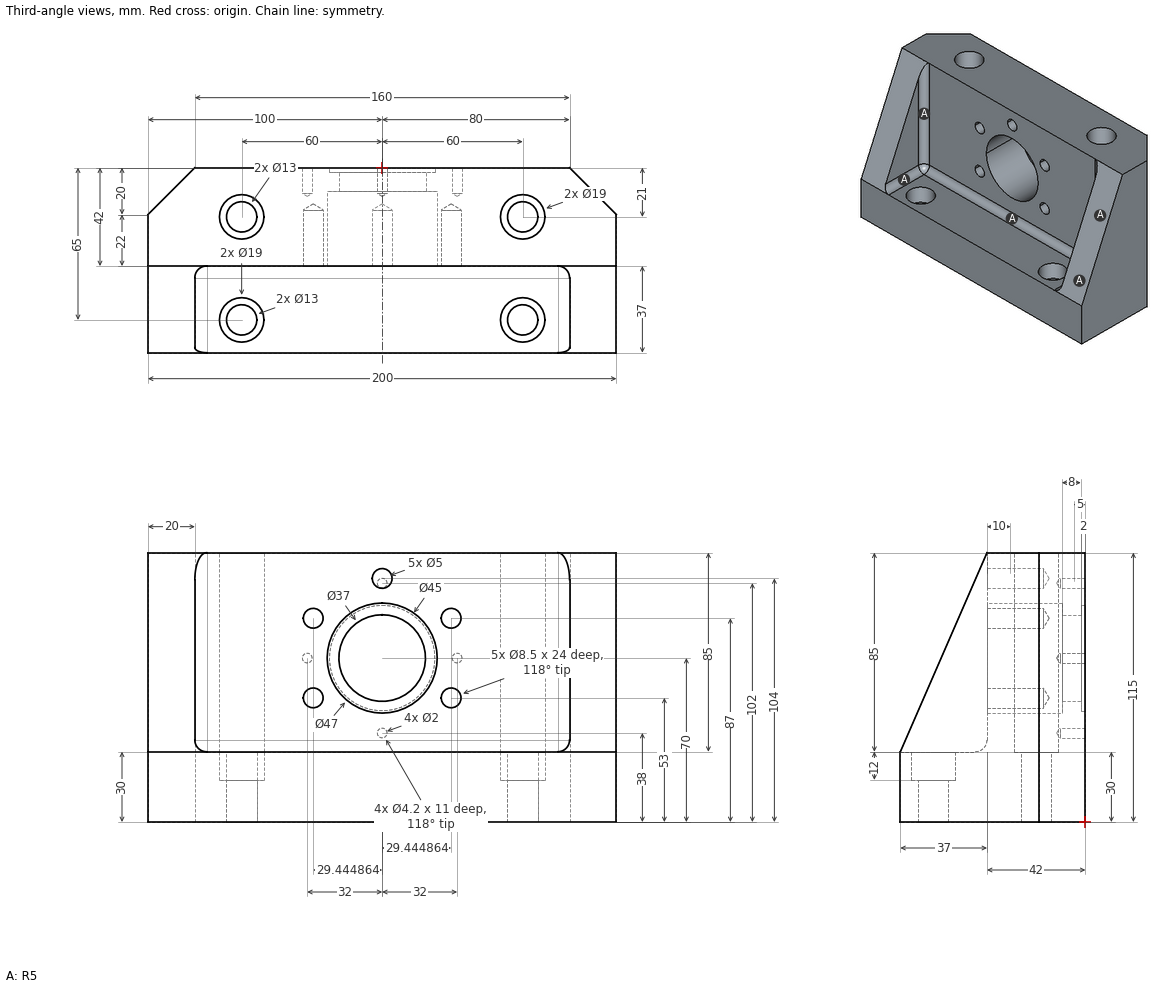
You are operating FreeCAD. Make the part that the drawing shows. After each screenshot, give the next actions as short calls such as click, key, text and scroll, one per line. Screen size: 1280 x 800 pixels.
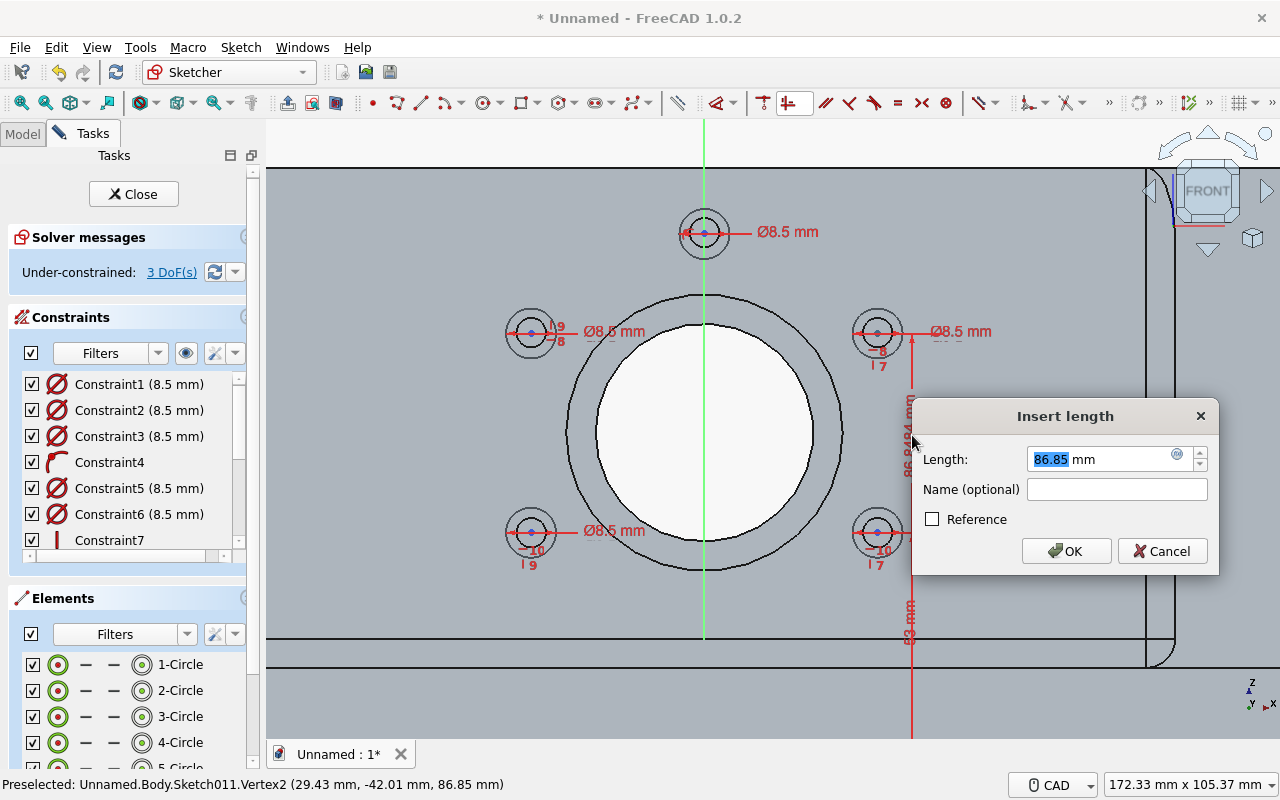
text(87)
key(Return)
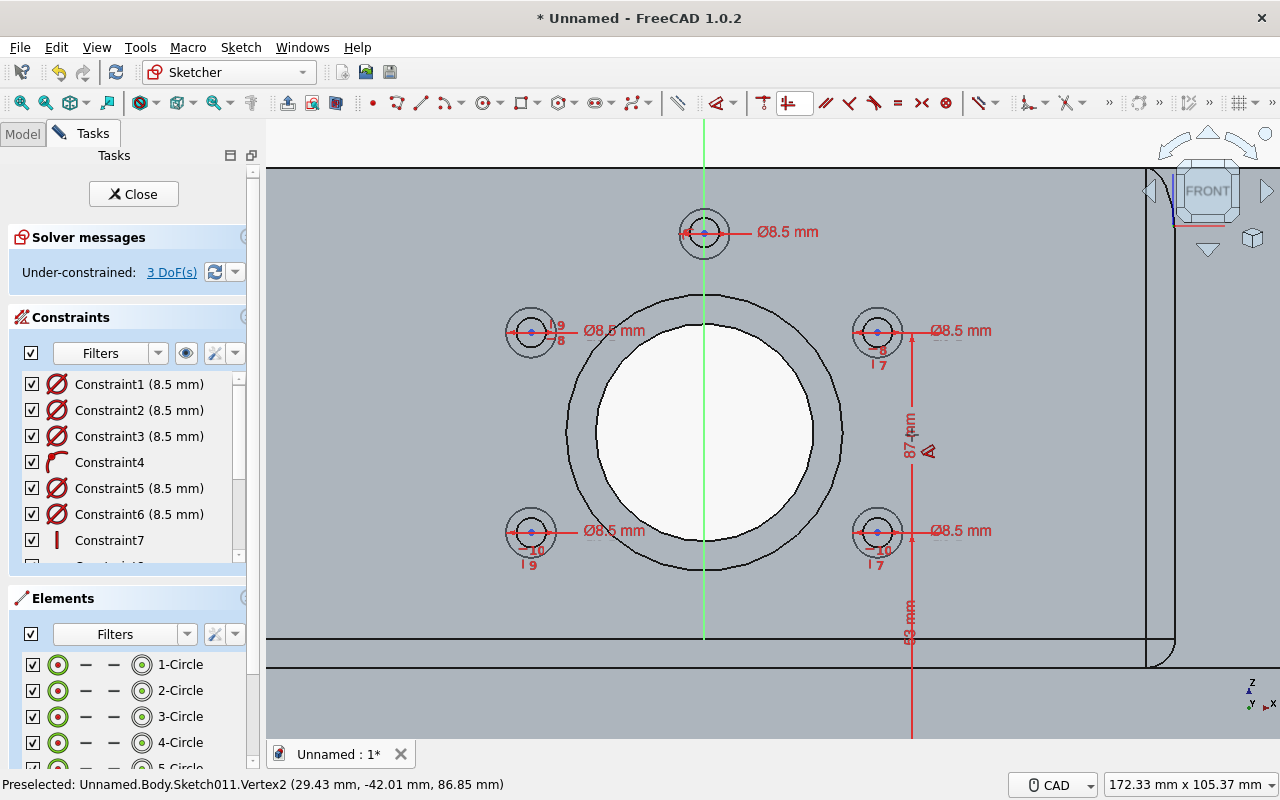
click(704, 234)
click(738, 472)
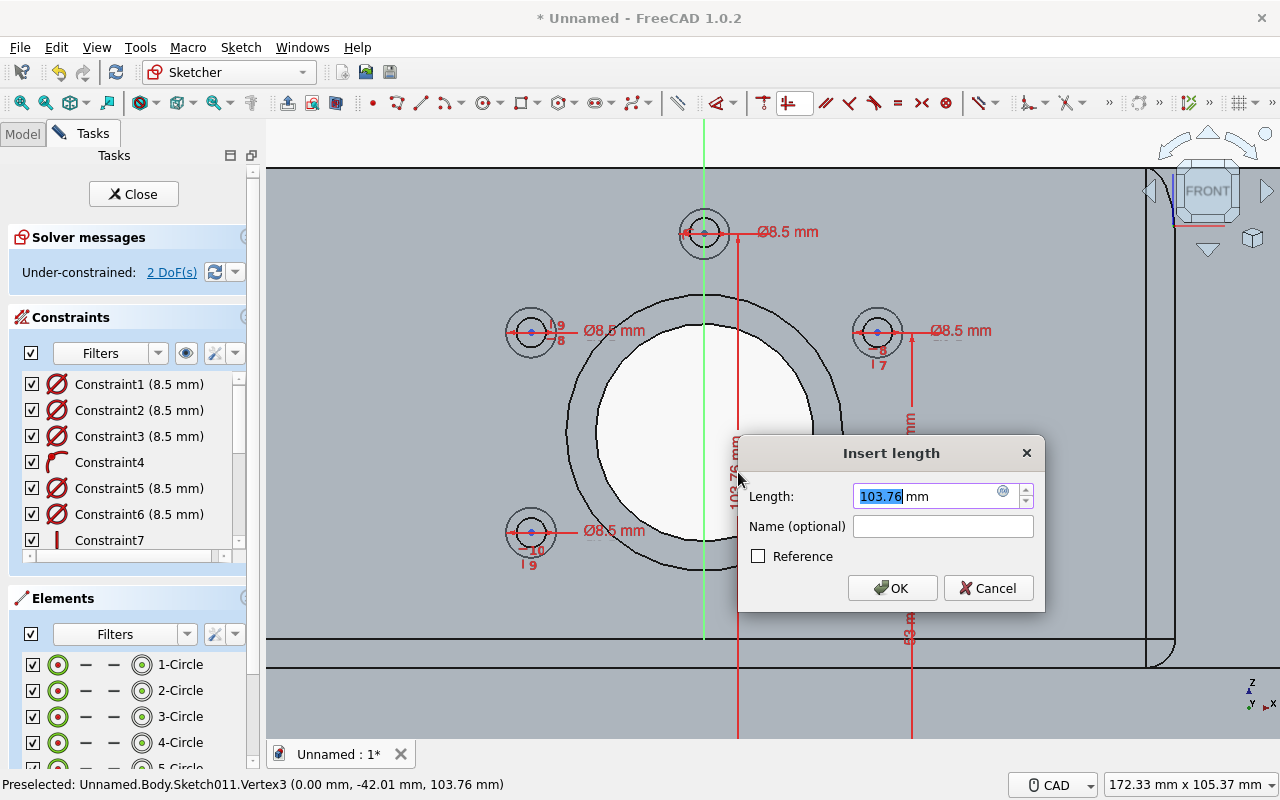
text(104)
key(Return)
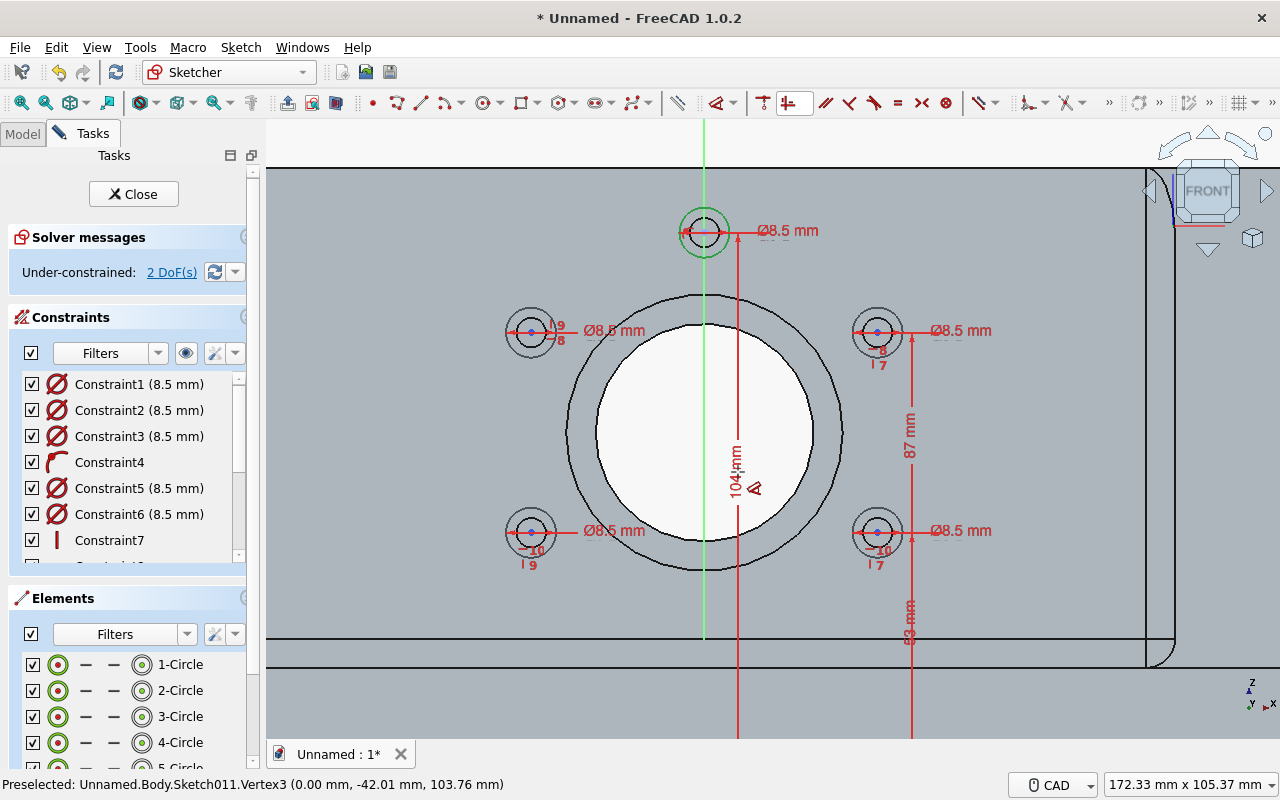
click(878, 533)
click(791, 499)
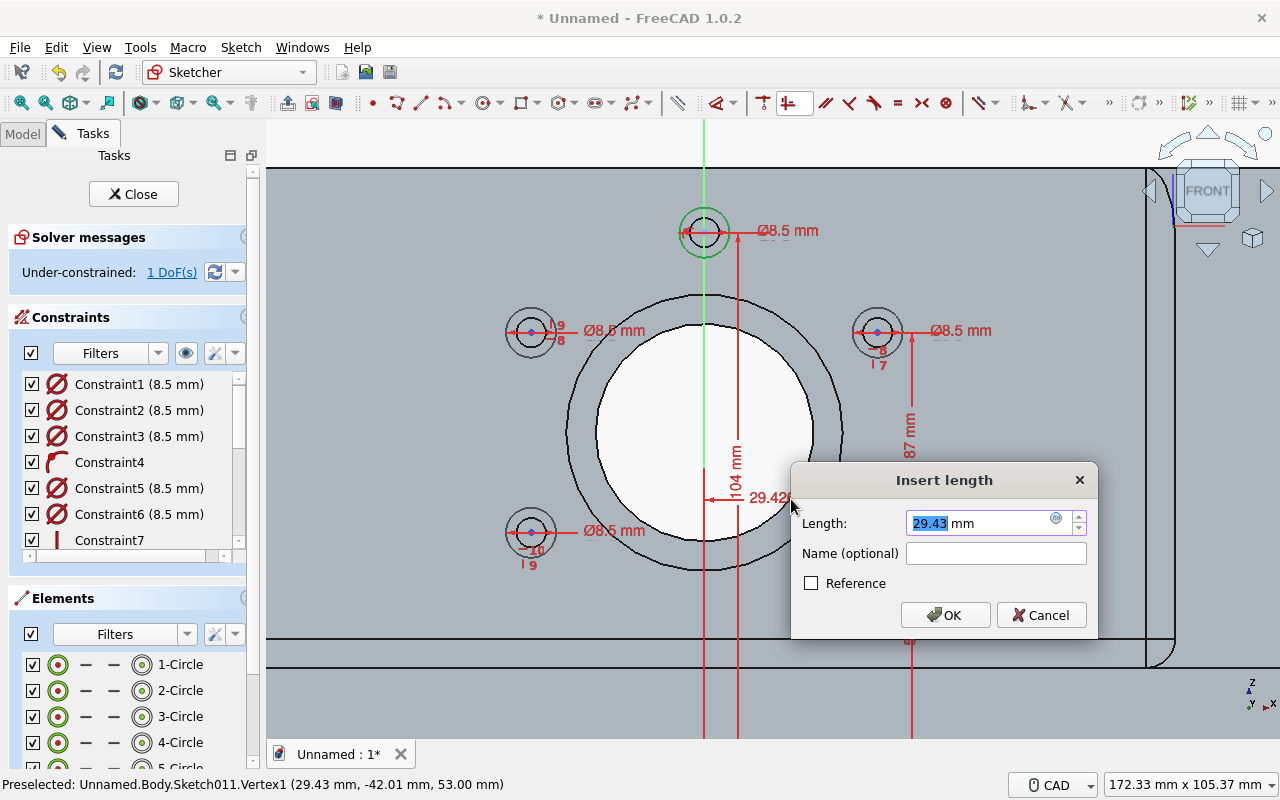
text(29.444864)
key(Return)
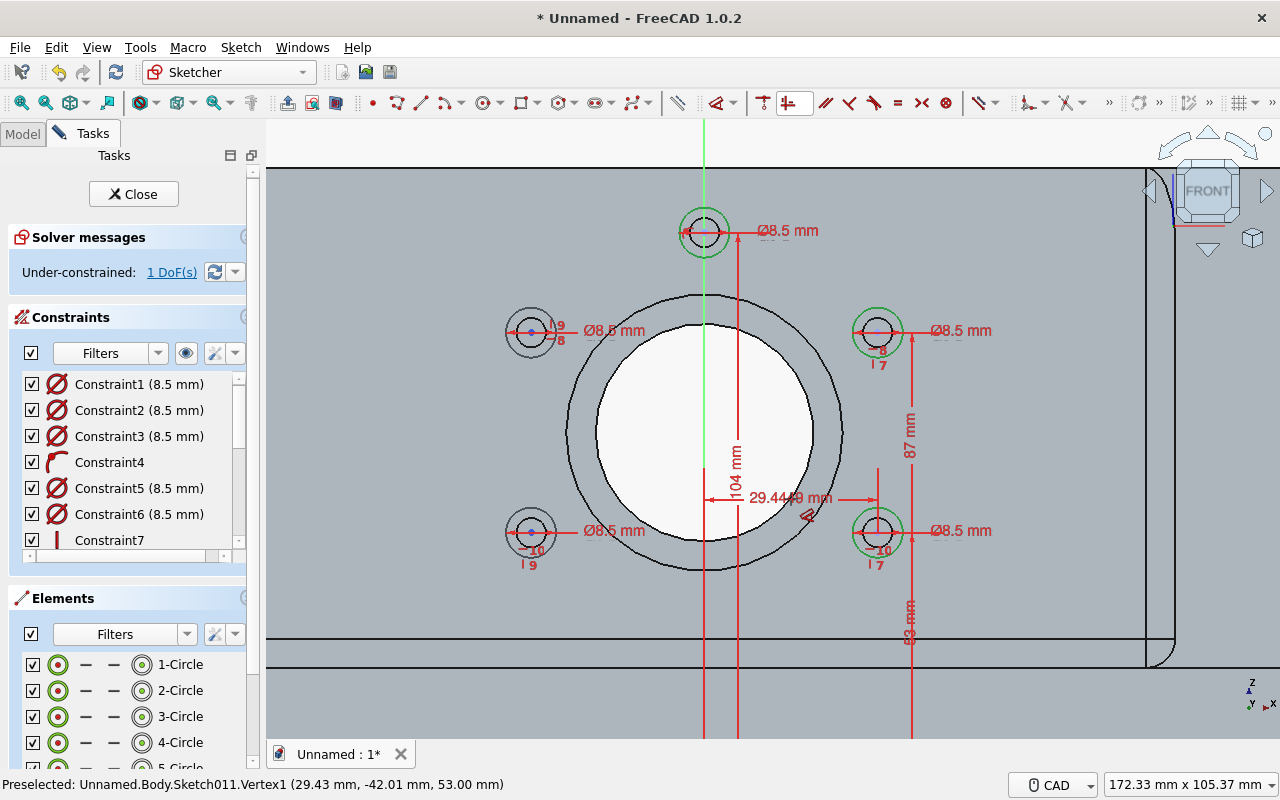
click(531, 333)
click(618, 299)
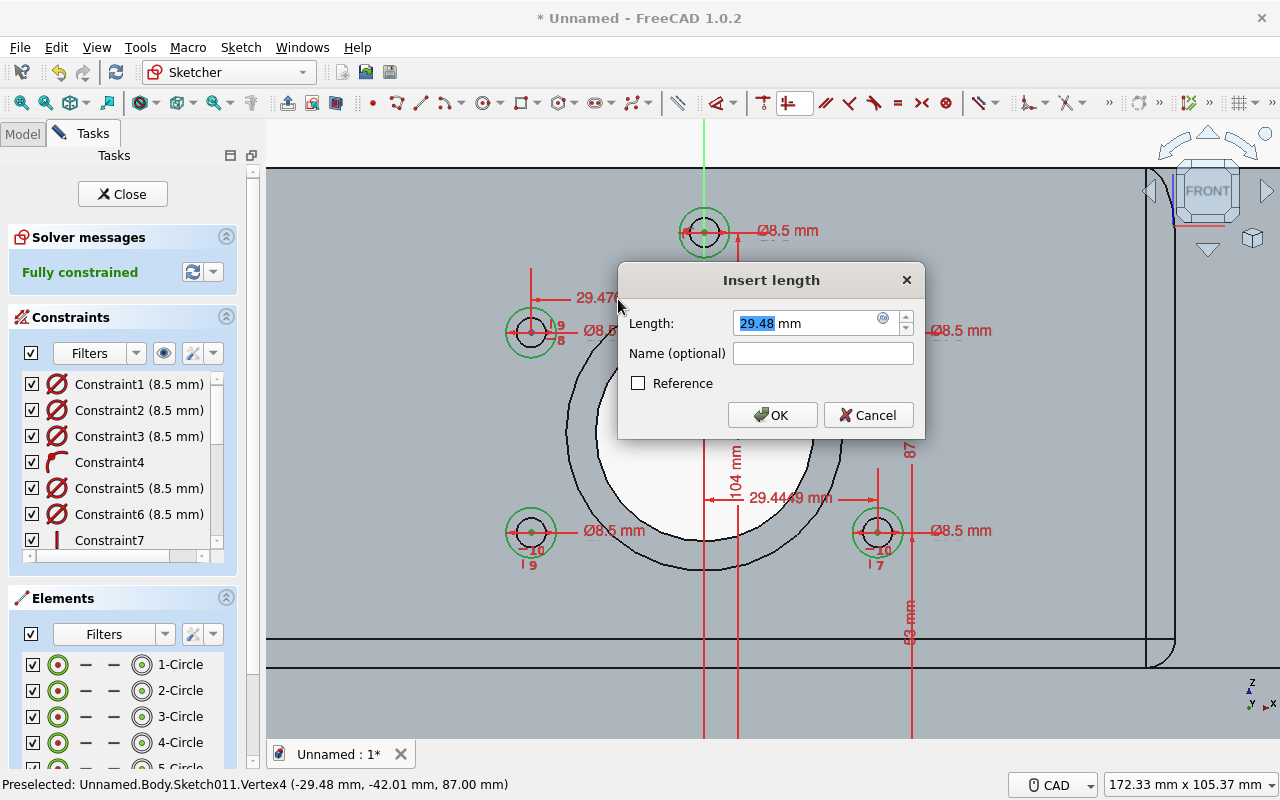
text(29.444864)
key(Return)
key(Escape)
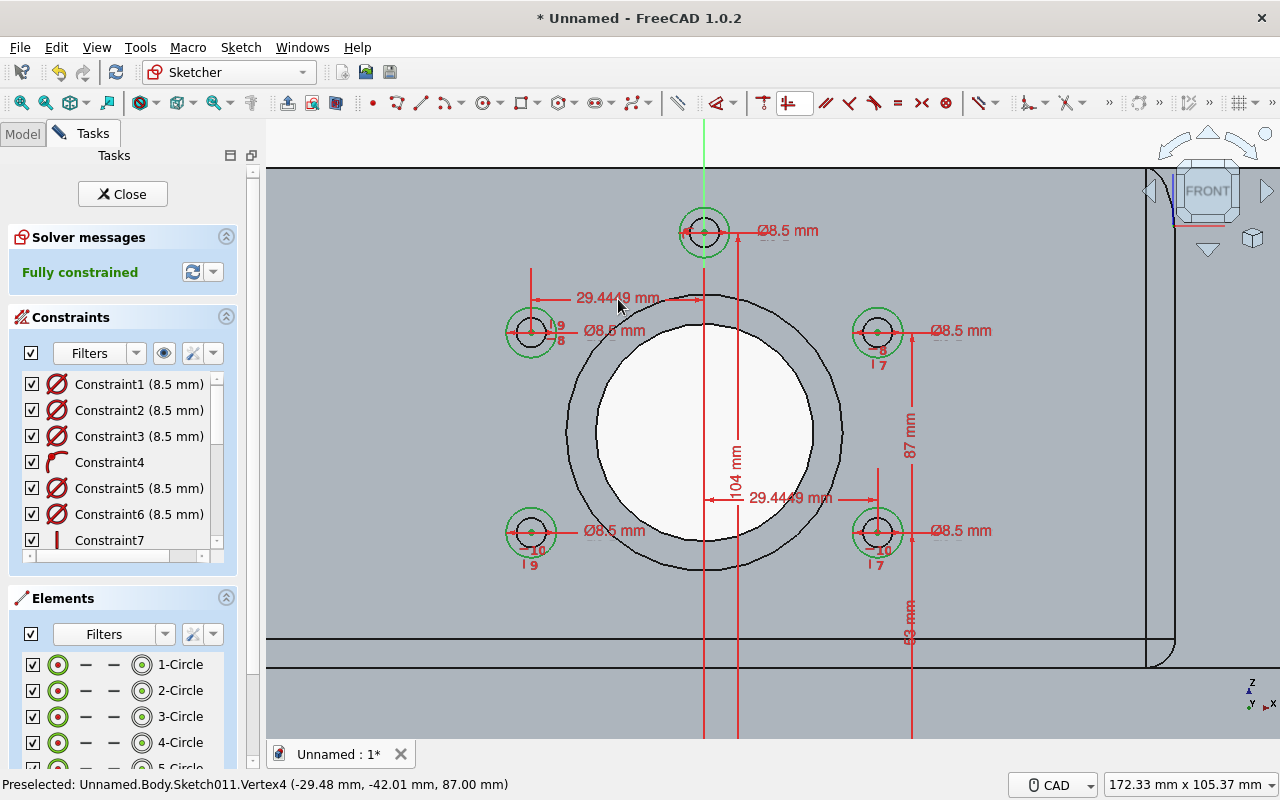
click(123, 194)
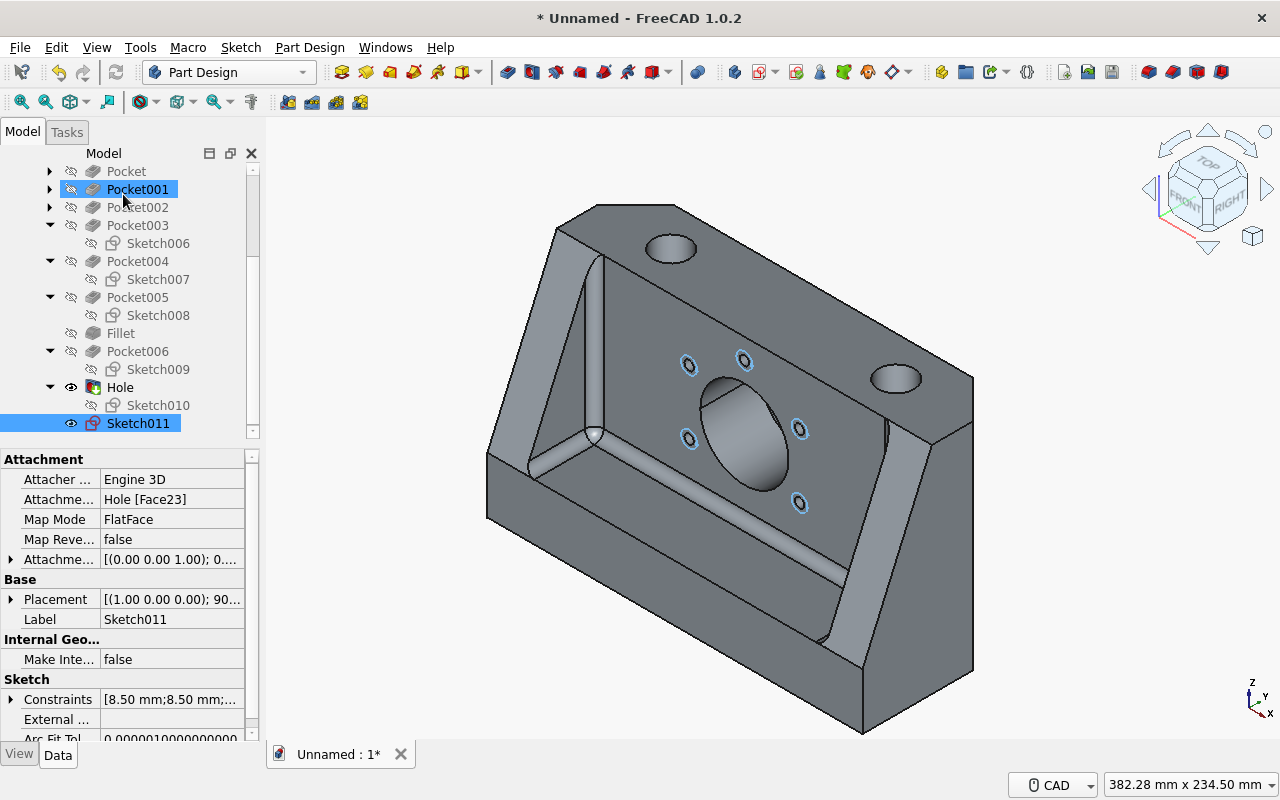
click(532, 72)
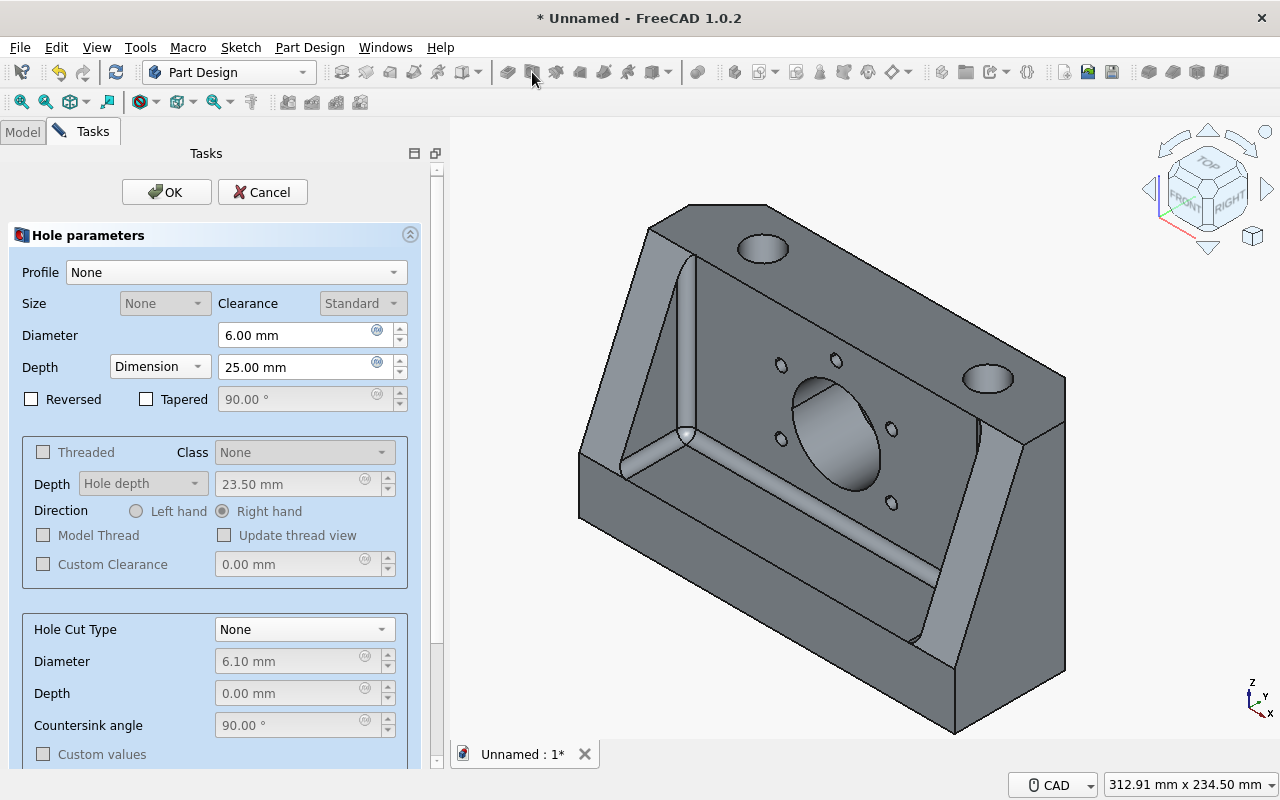
triple_click(305, 335)